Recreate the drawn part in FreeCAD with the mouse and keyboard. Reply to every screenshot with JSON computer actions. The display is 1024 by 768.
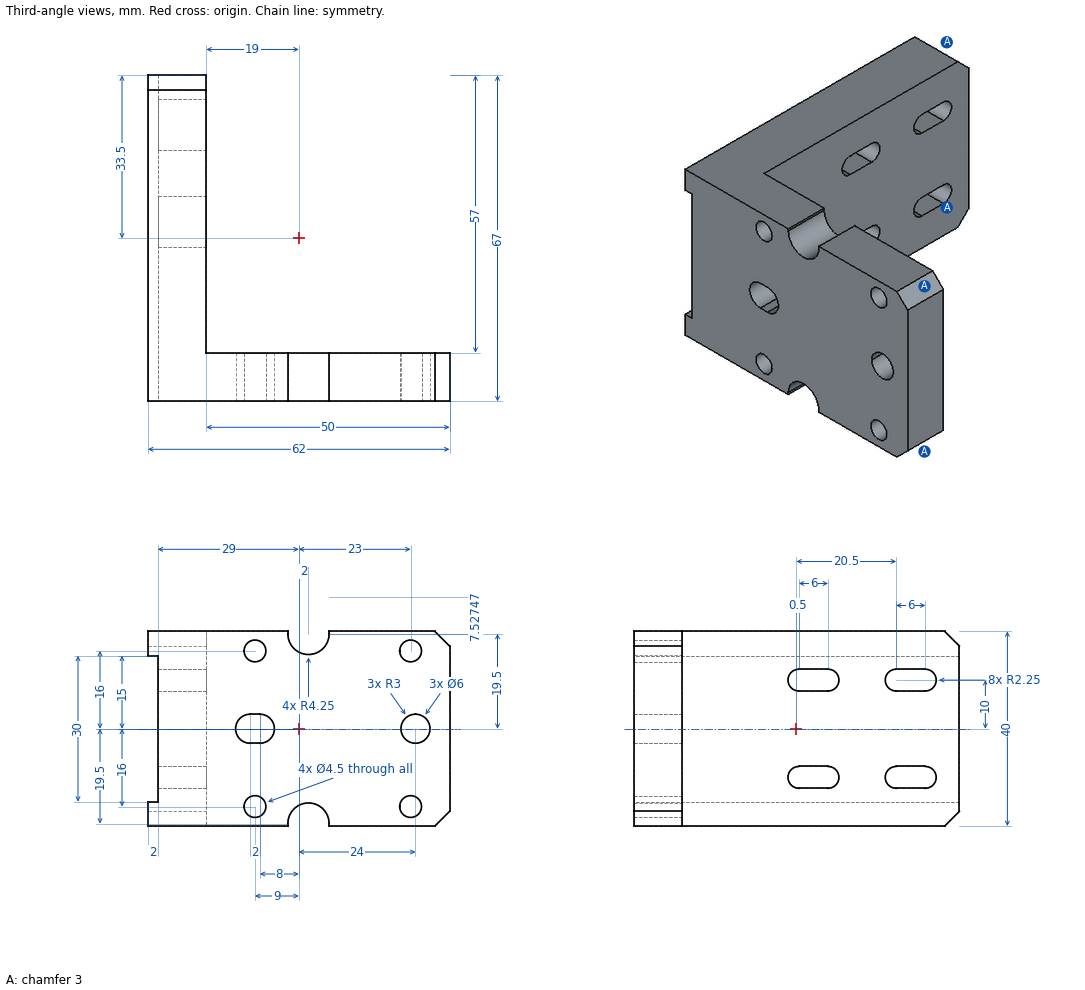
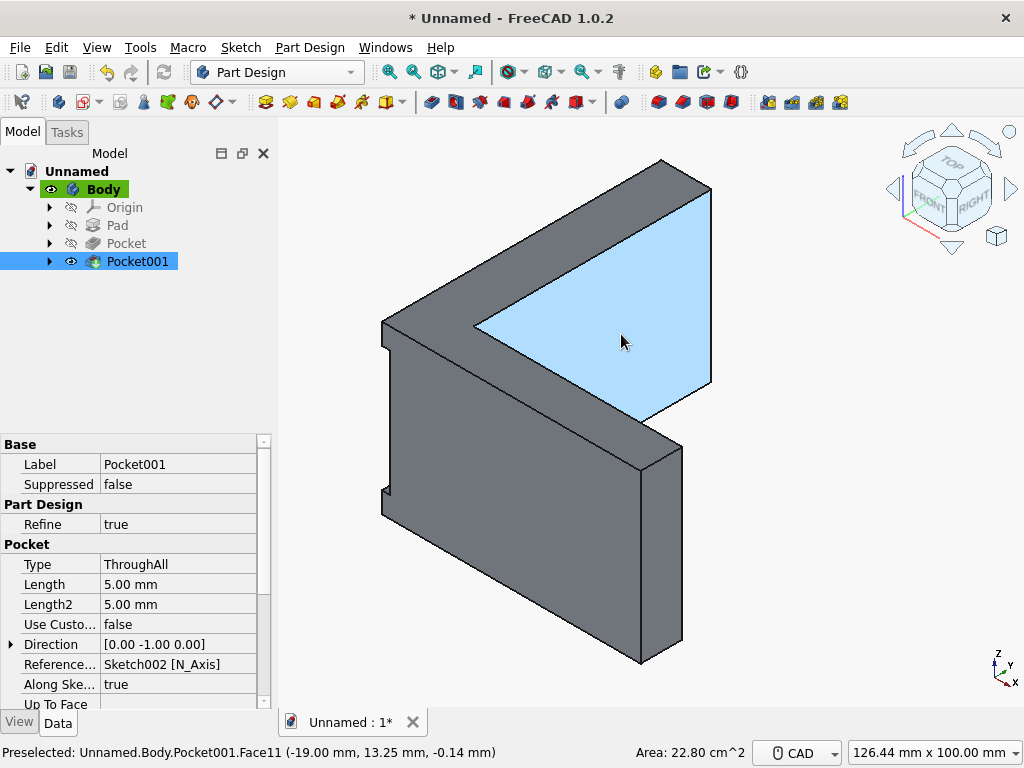
{"action": "left_click", "coordinate": [84, 102]}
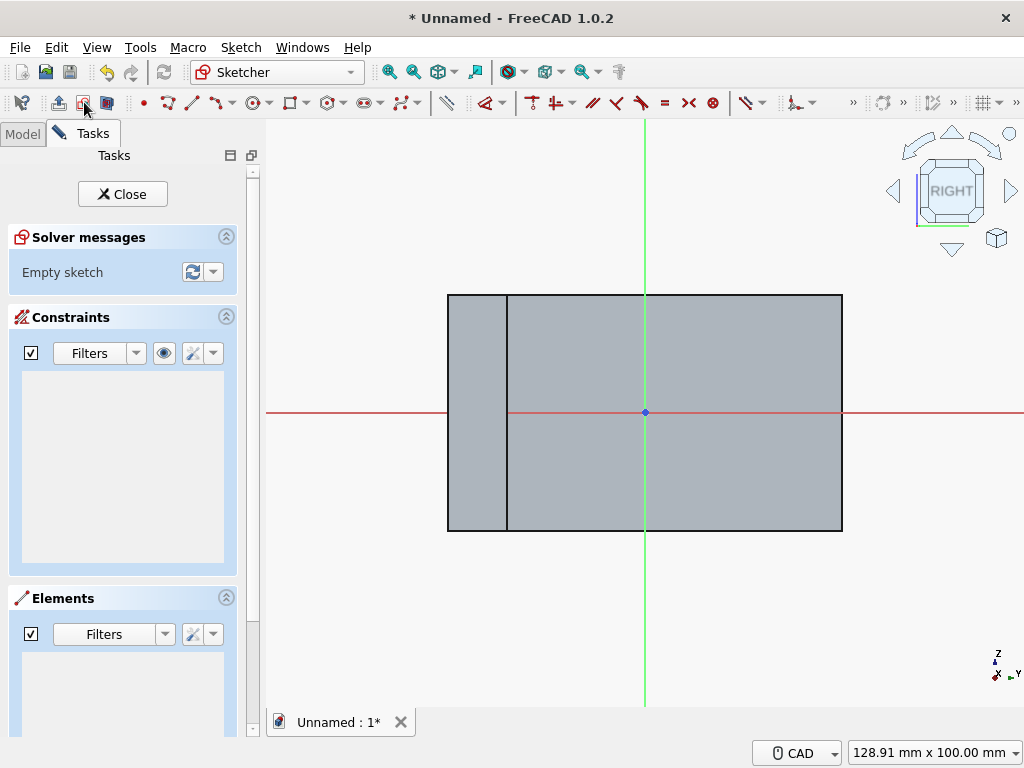
{"action": "left_click", "coordinate": [108, 104]}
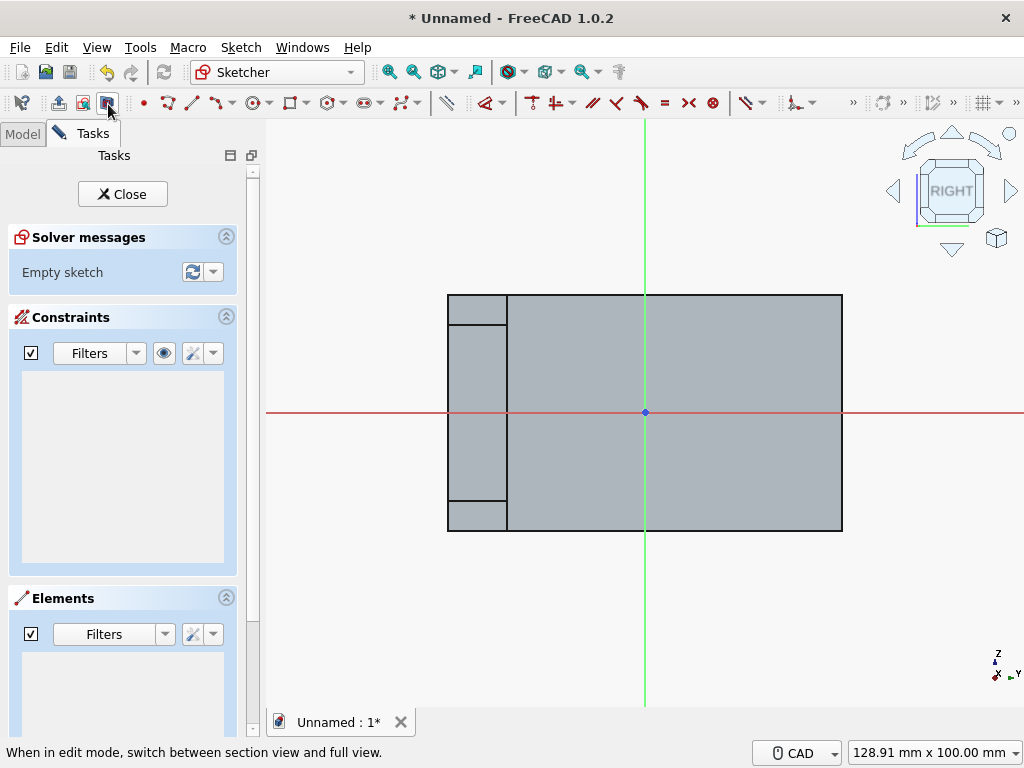
{"action": "scroll", "coordinate": [845, 413], "scroll_direction": "up", "scroll_amount": 4}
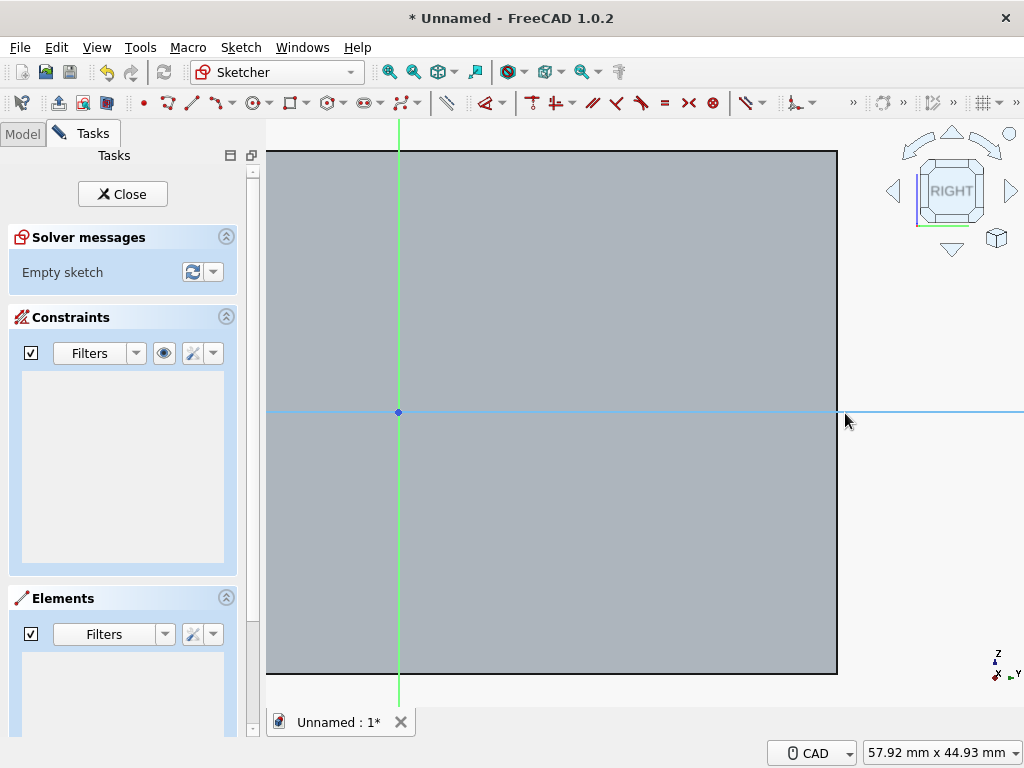
{"action": "left_click", "coordinate": [364, 104]}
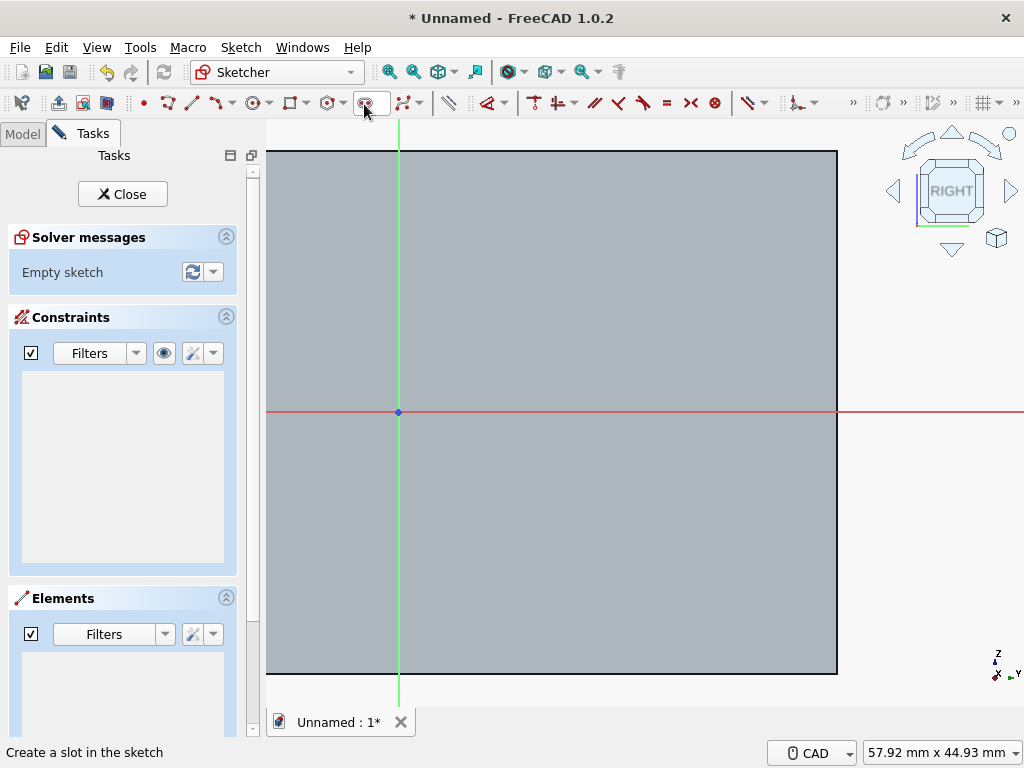
{"action": "left_click", "coordinate": [667, 282]}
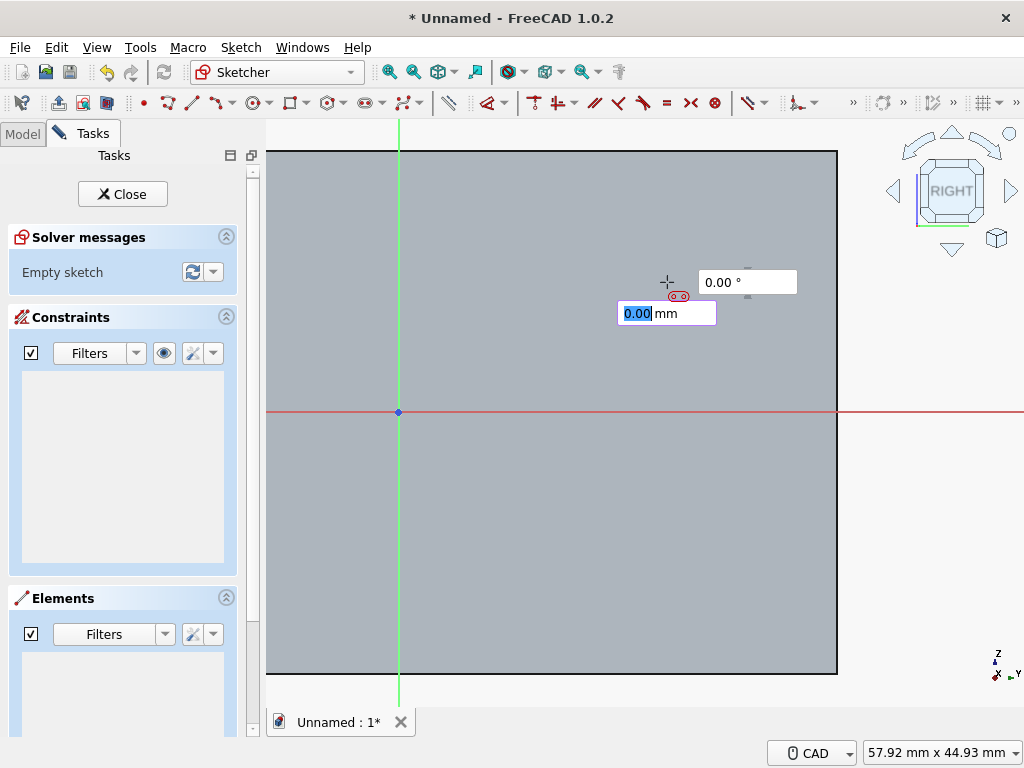
{"action": "left_click", "coordinate": [746, 282]}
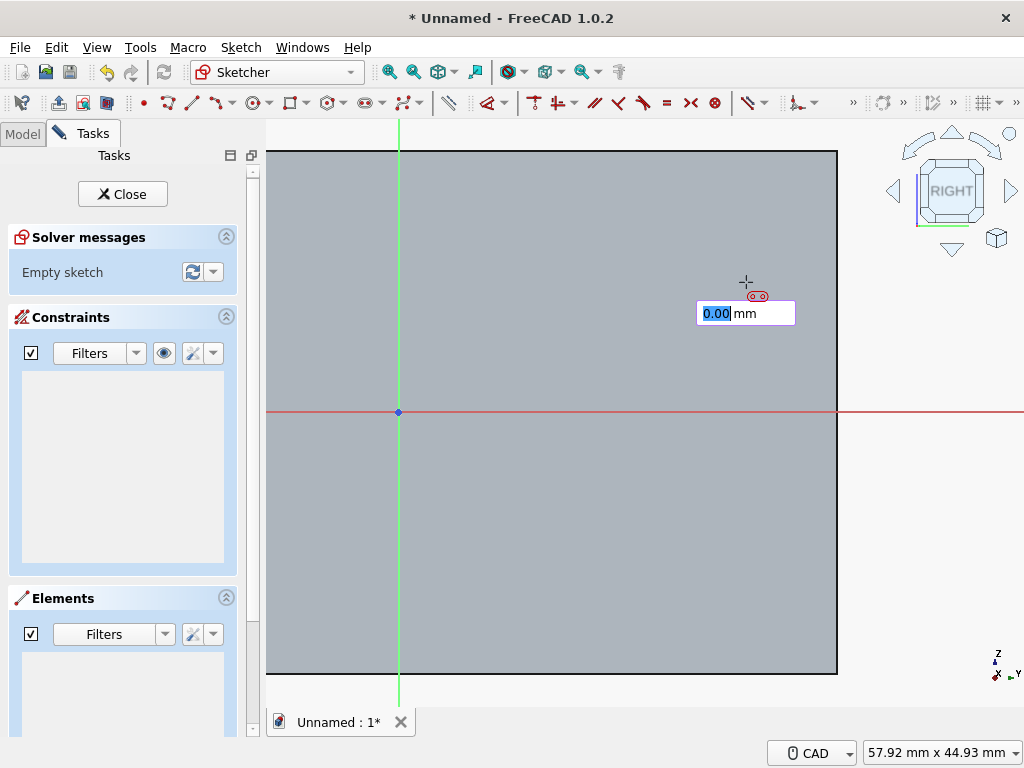
{"action": "left_click", "coordinate": [706, 311]}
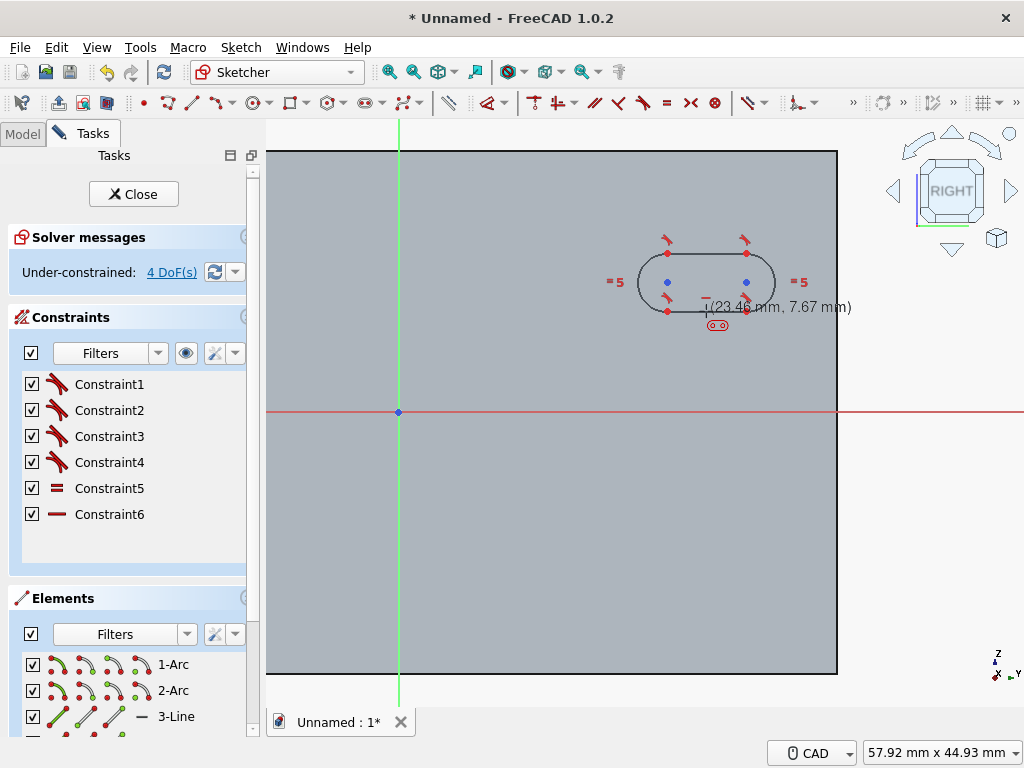
{"action": "scroll", "coordinate": [405, 282], "scroll_direction": "up", "scroll_amount": 5}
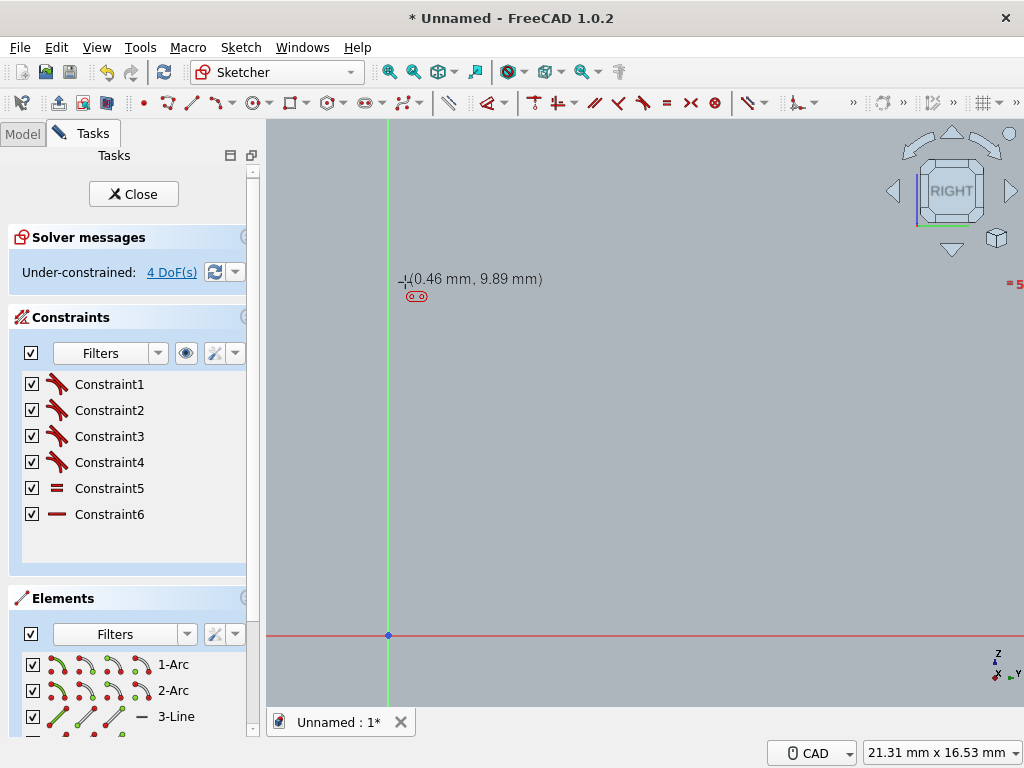
{"action": "left_click", "coordinate": [406, 280]}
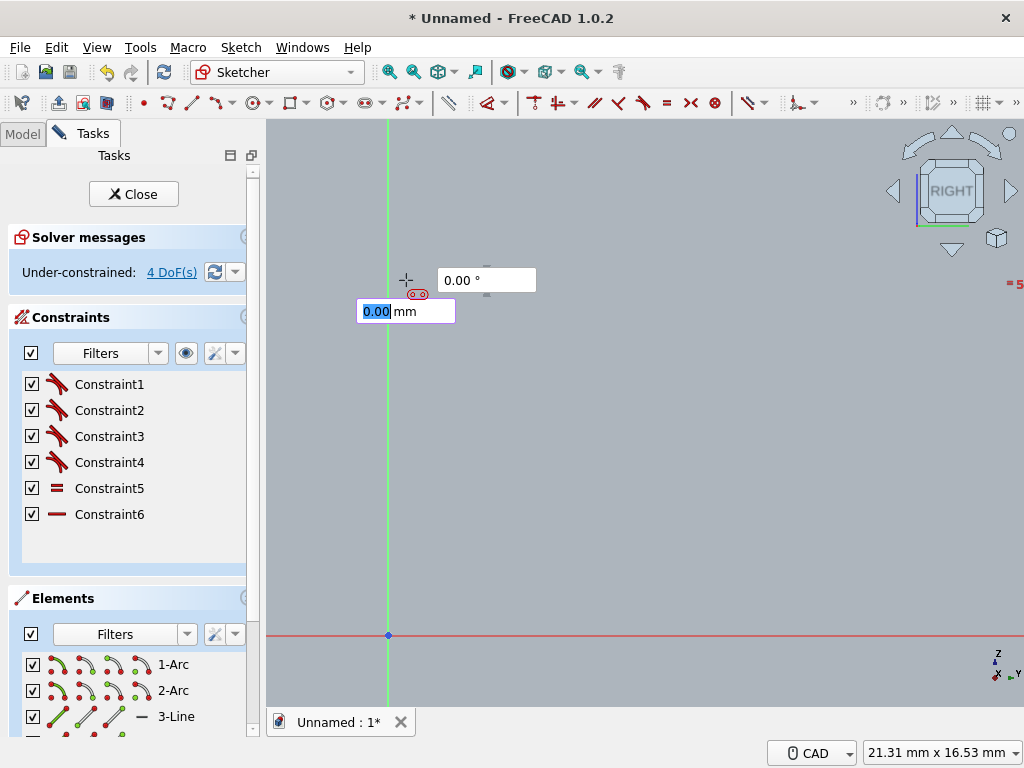
{"action": "left_click", "coordinate": [619, 280]}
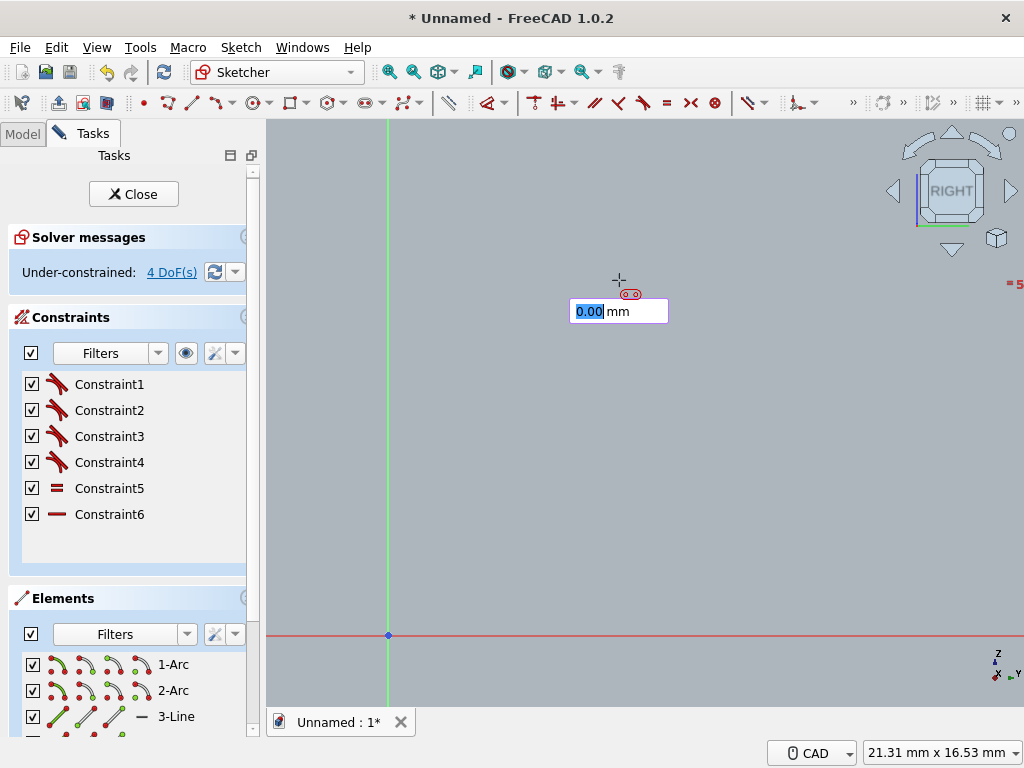
{"action": "left_click", "coordinate": [513, 360]}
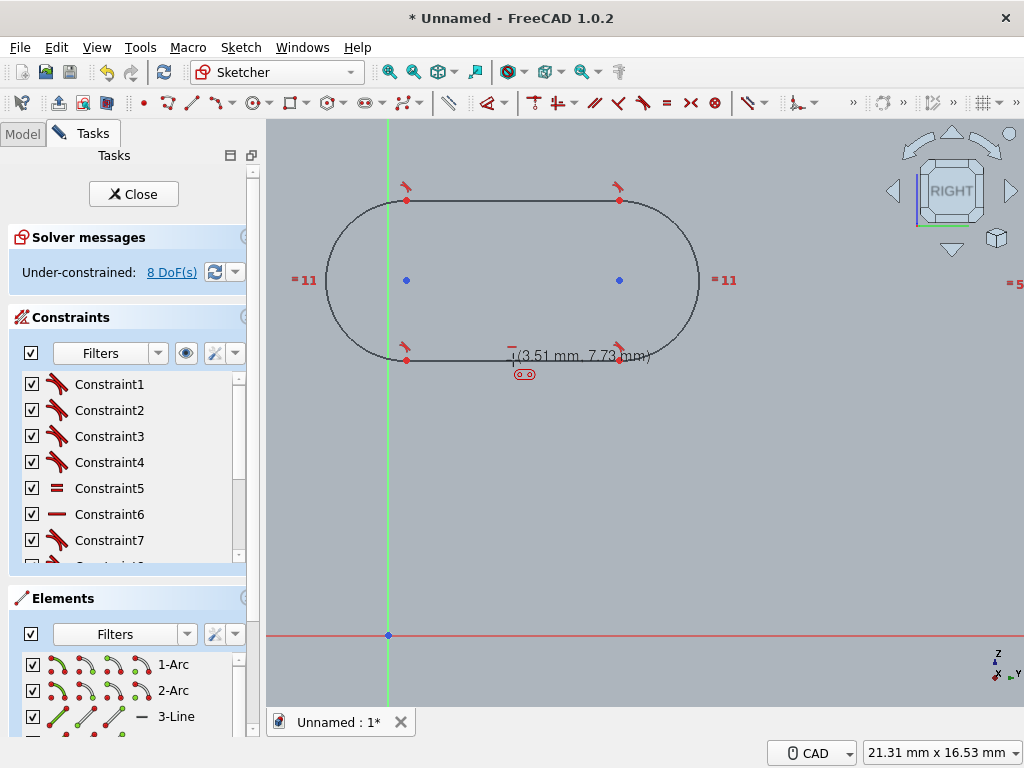
{"action": "scroll", "coordinate": [407, 283], "scroll_direction": "down", "scroll_amount": 5}